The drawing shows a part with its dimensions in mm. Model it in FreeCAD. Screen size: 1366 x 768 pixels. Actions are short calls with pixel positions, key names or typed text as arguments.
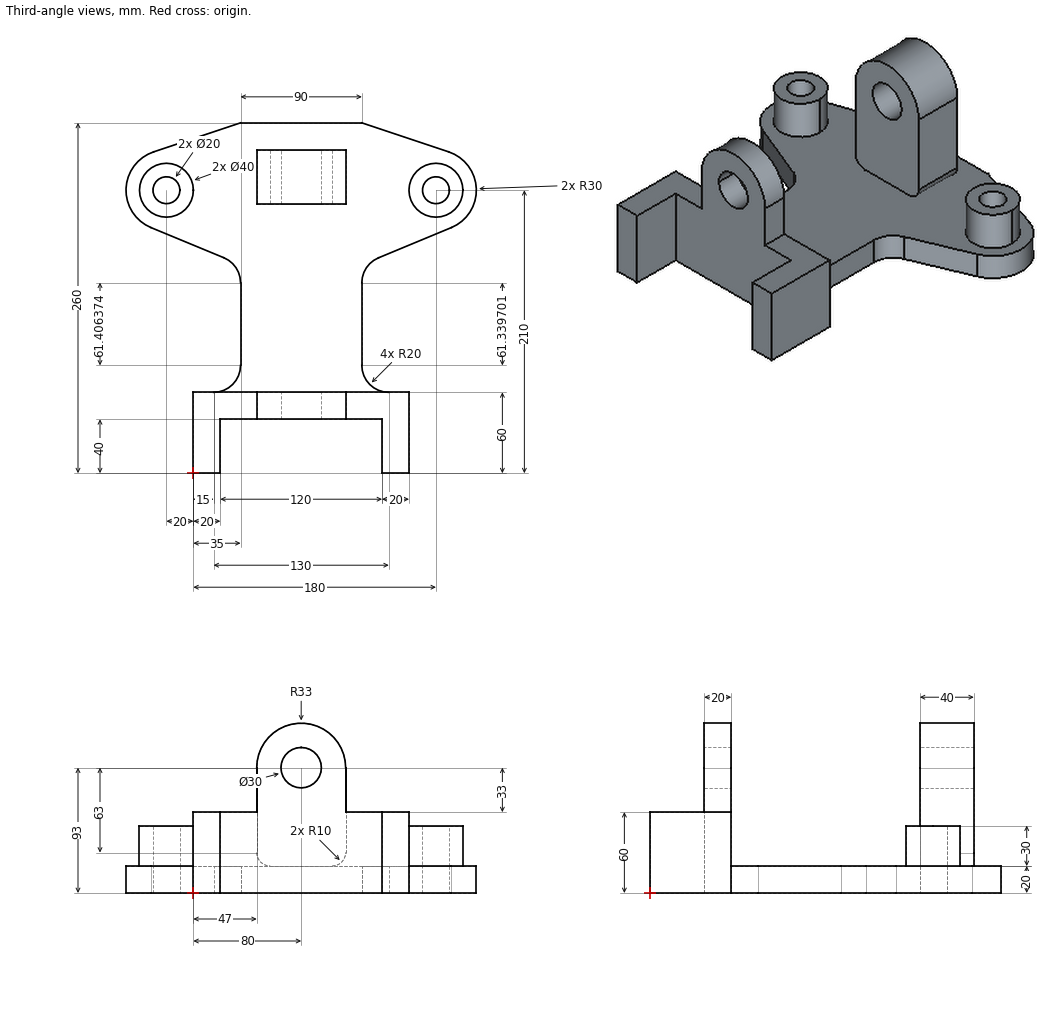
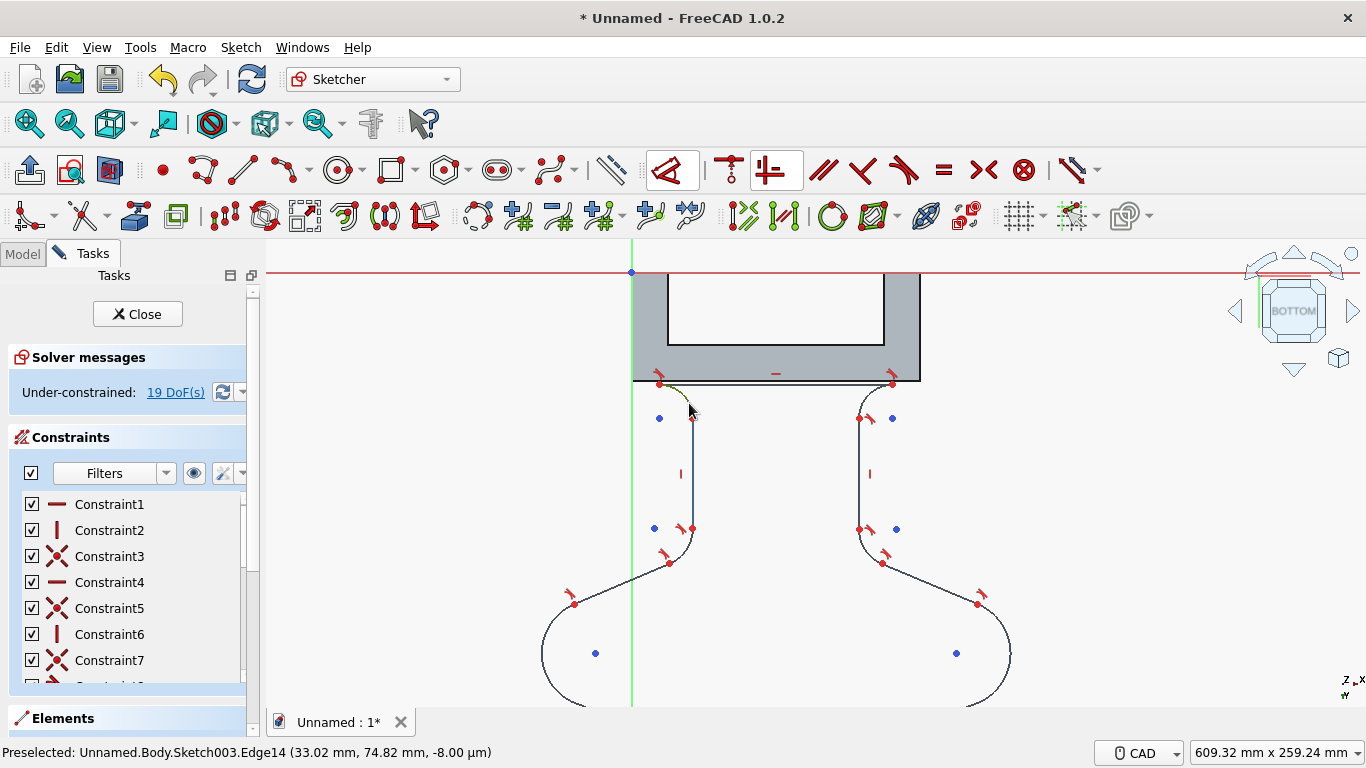
click(904, 170)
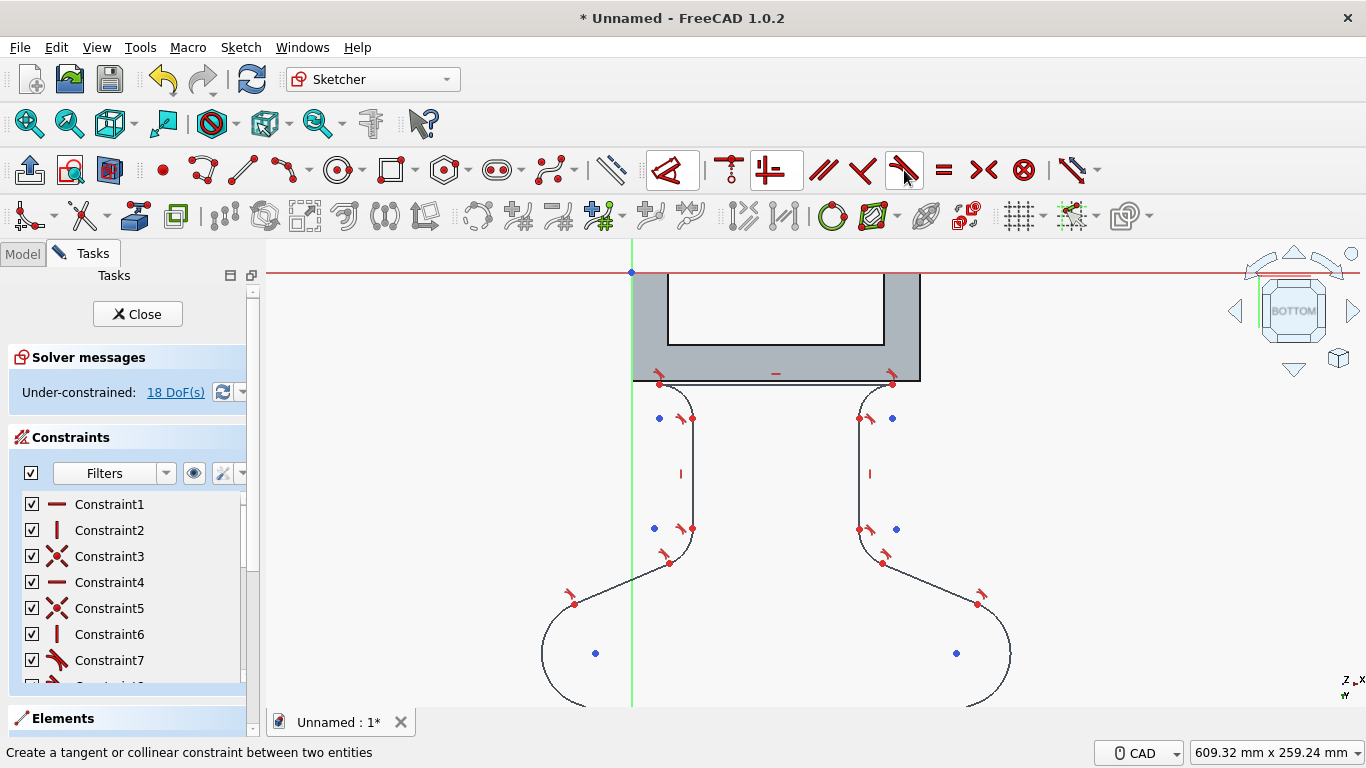
click(863, 403)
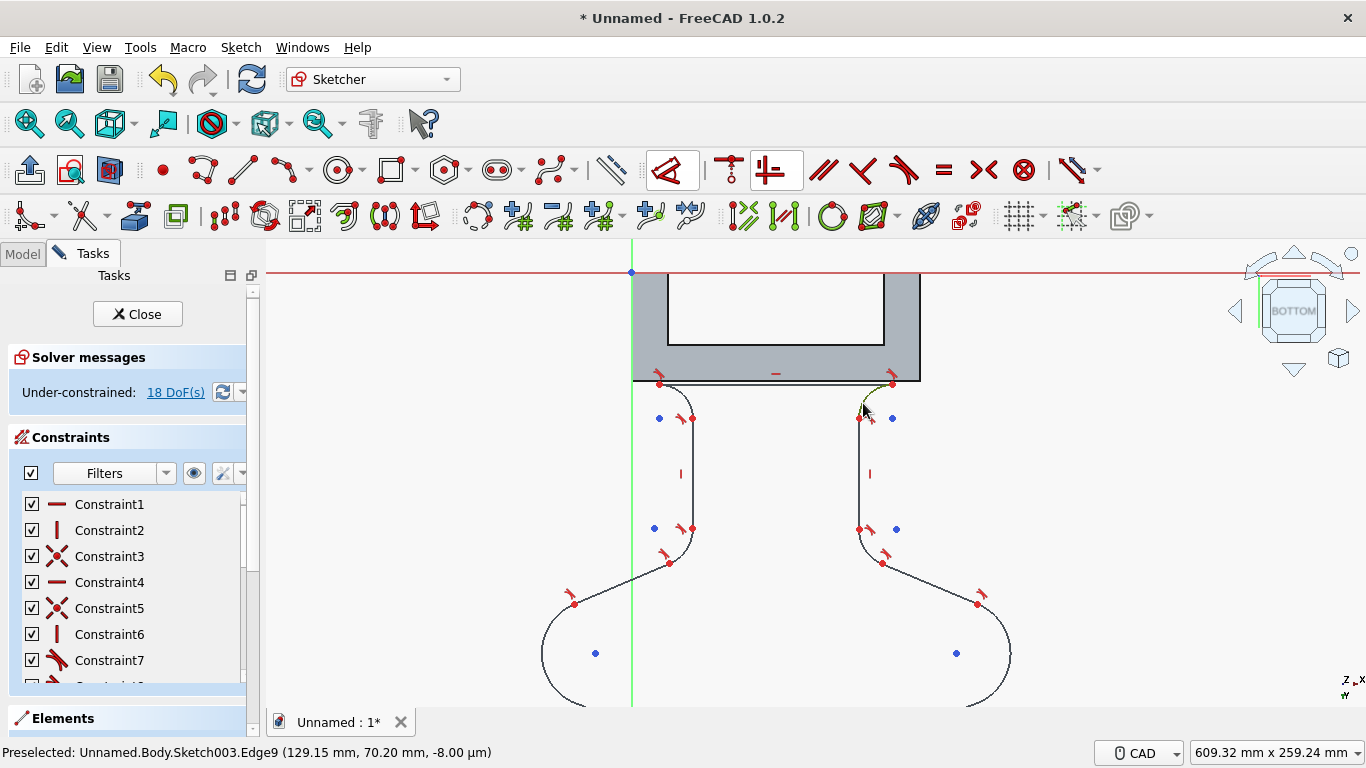
click(861, 542)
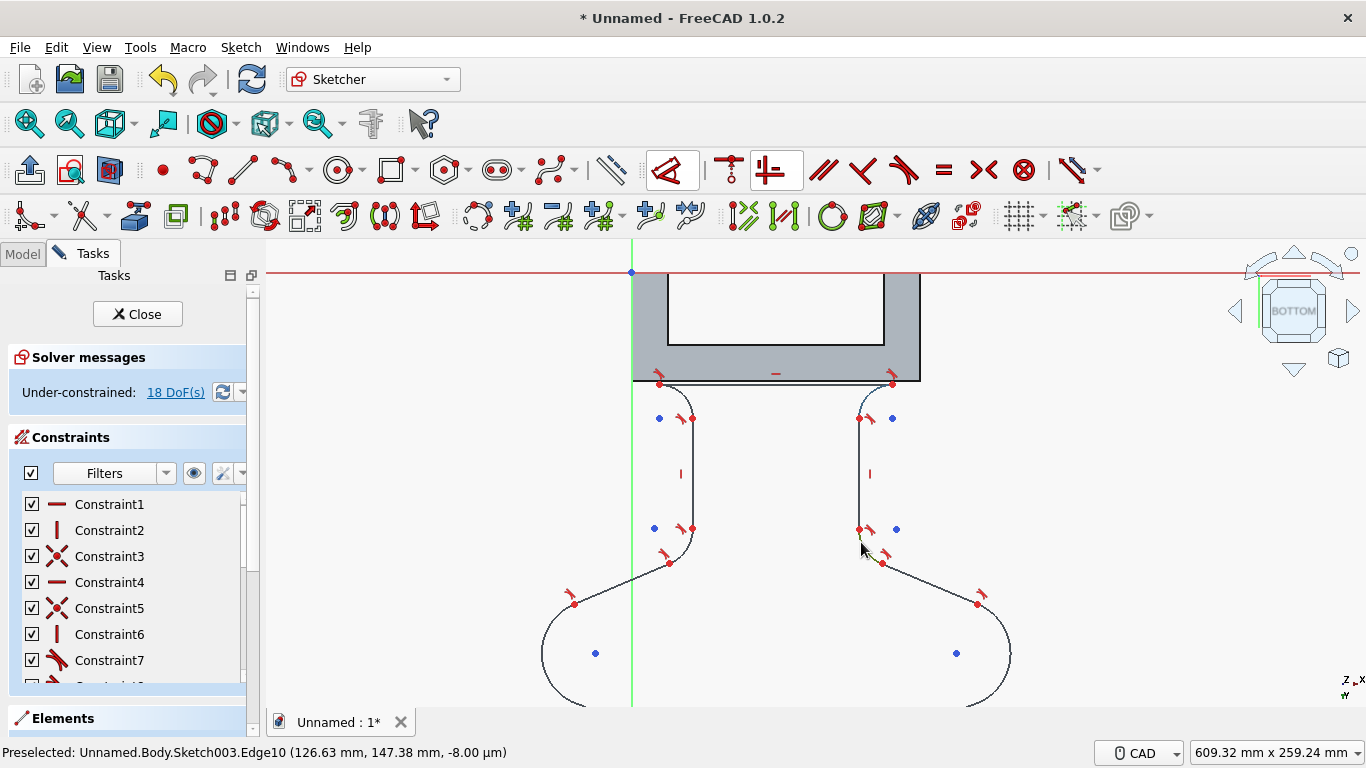
click(681, 557)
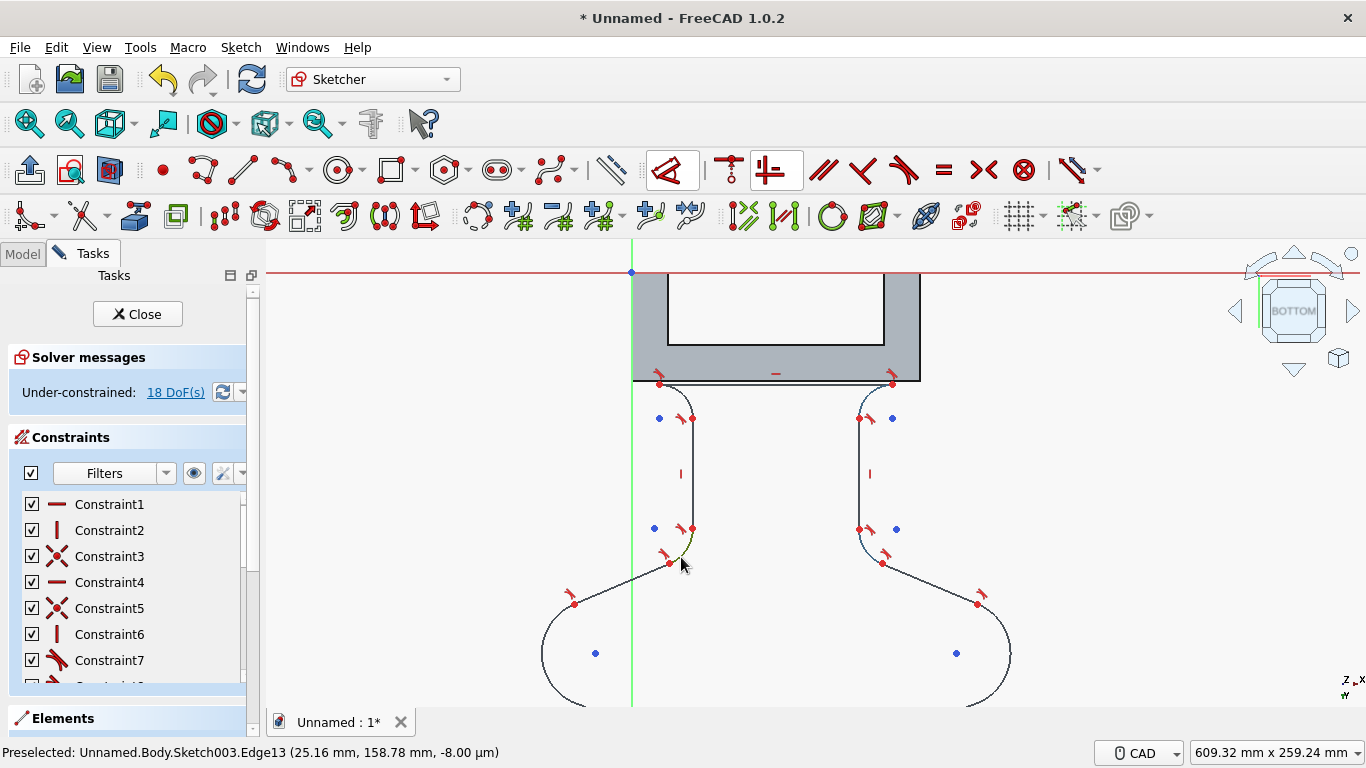
click(689, 403)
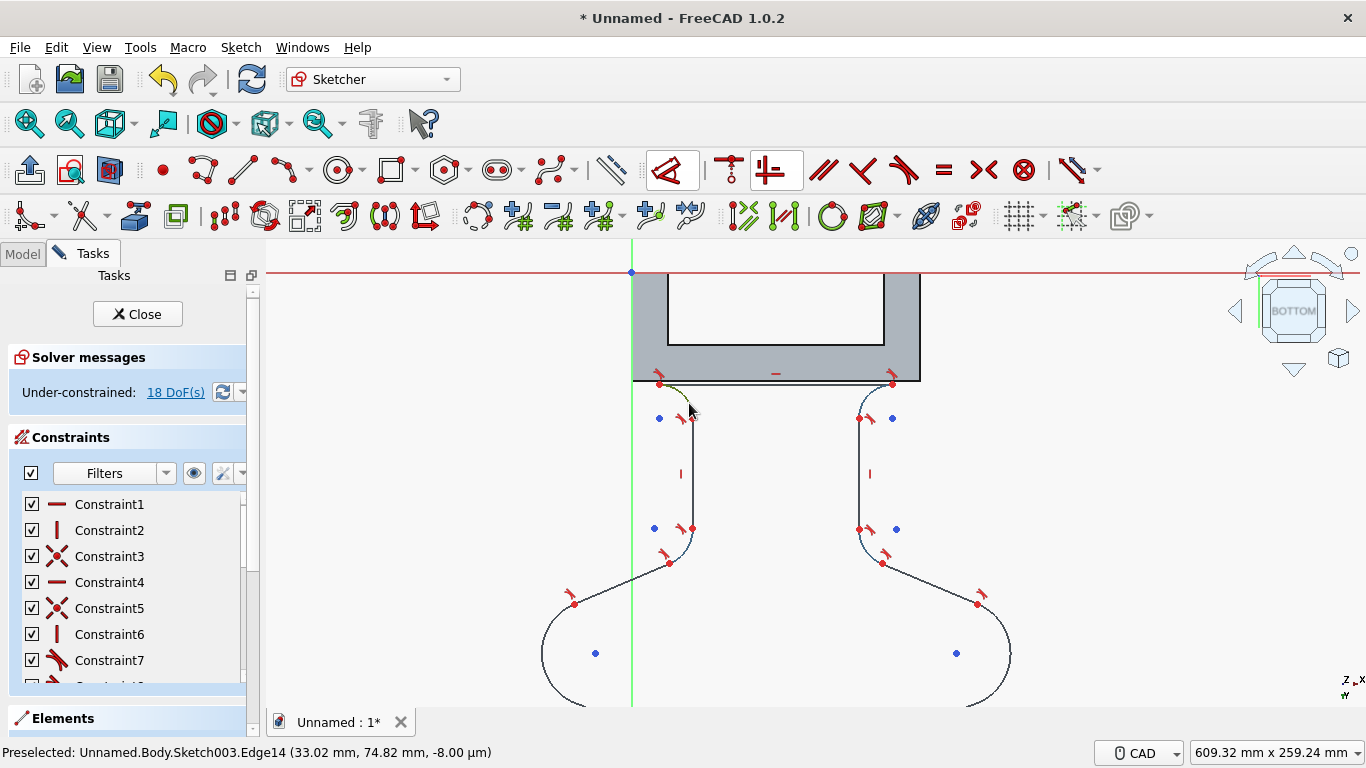
click(944, 170)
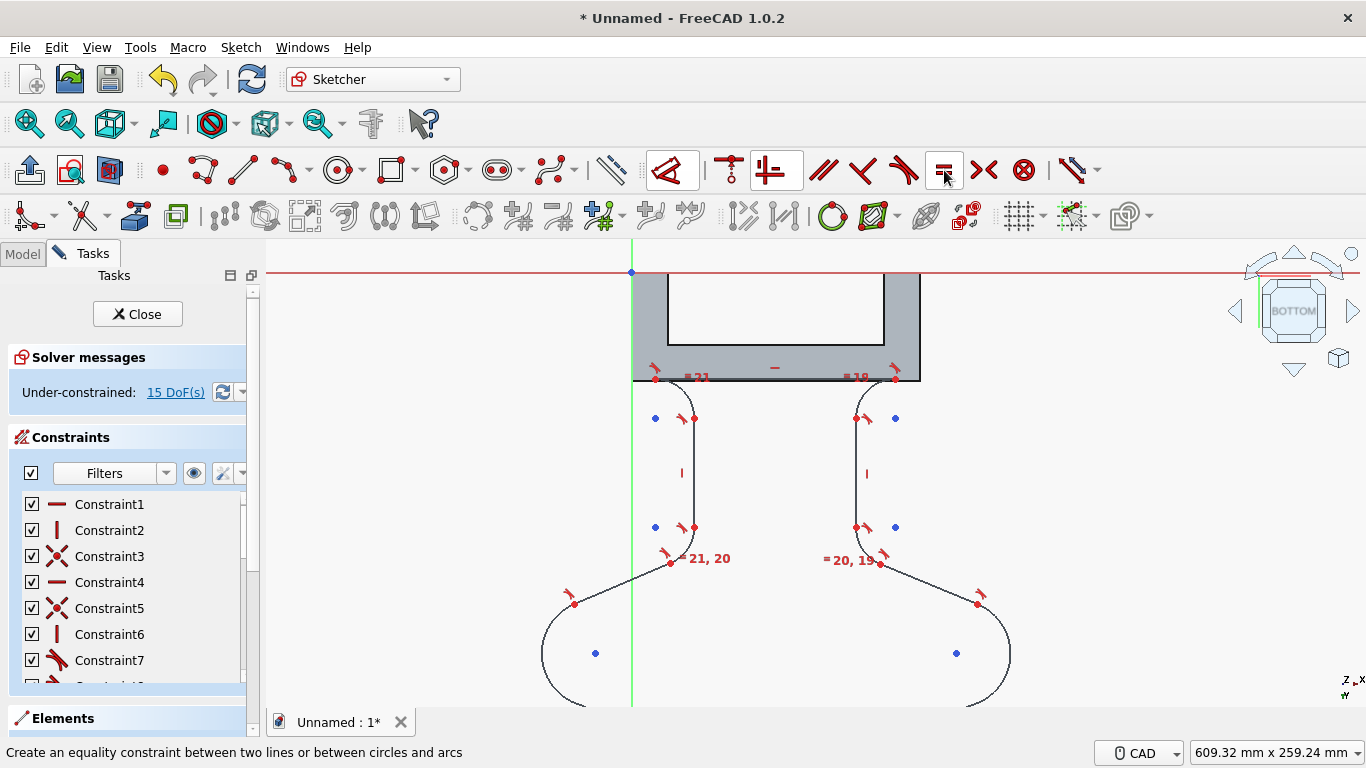
click(1005, 630)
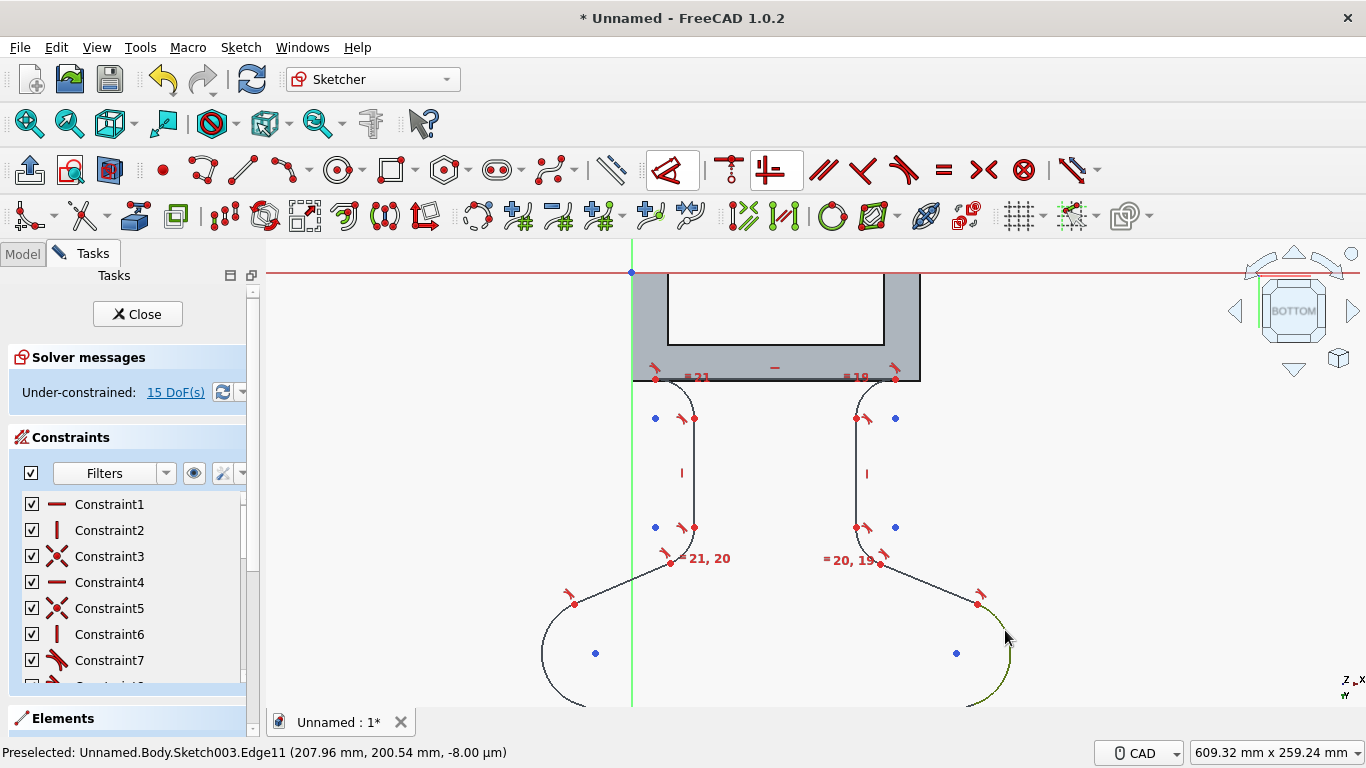
click(547, 630)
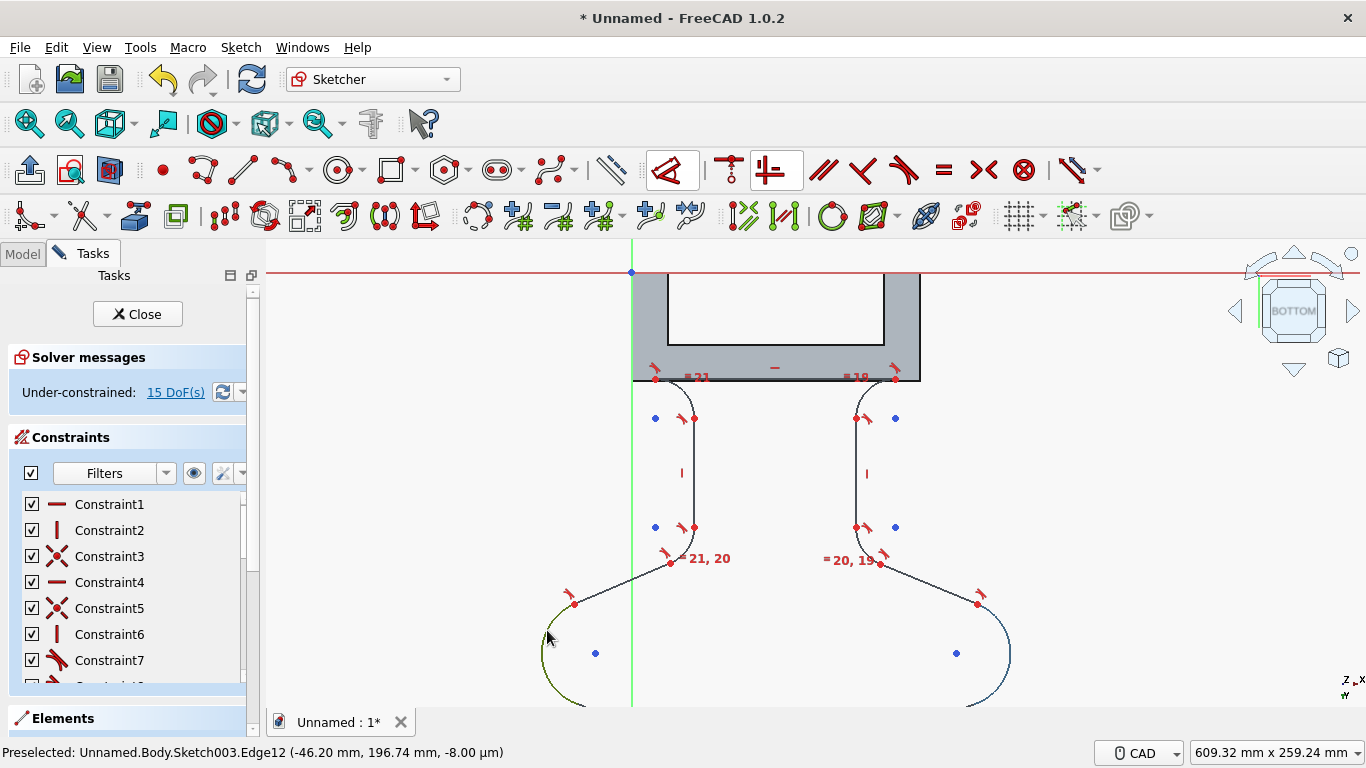
click(944, 170)